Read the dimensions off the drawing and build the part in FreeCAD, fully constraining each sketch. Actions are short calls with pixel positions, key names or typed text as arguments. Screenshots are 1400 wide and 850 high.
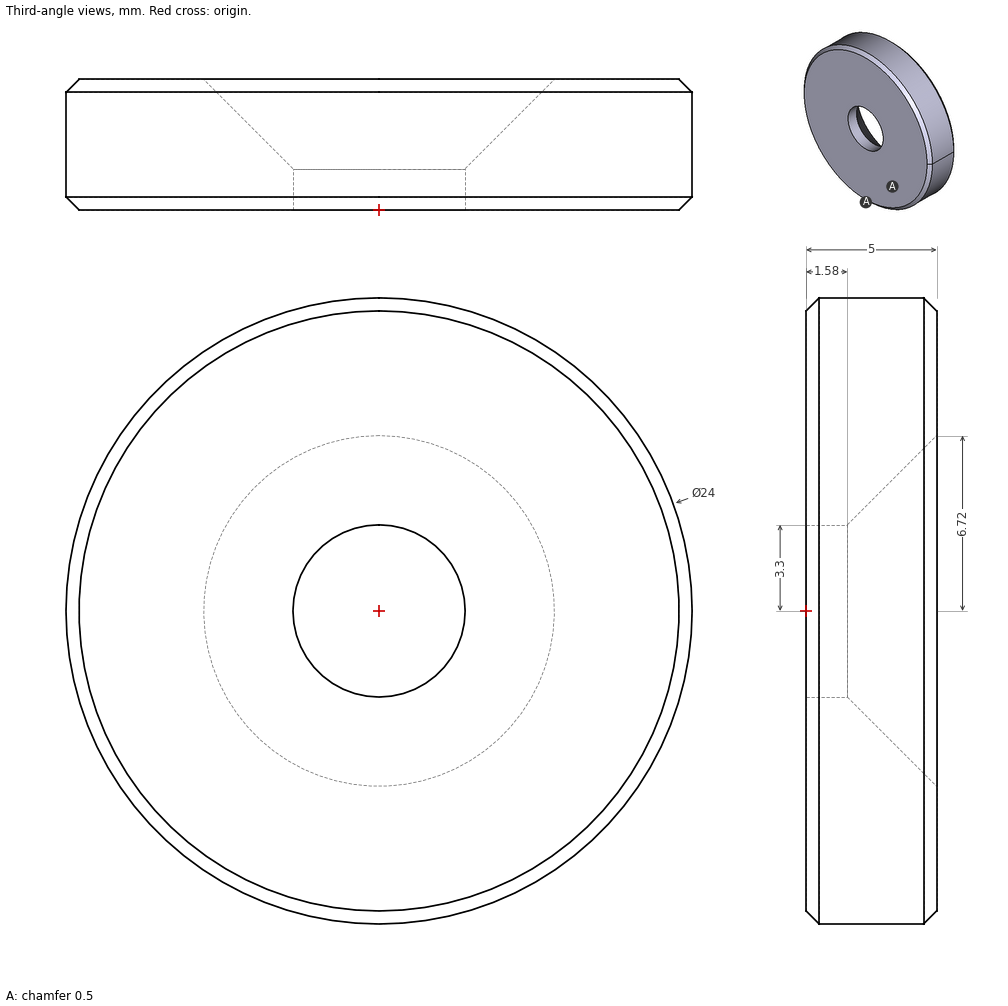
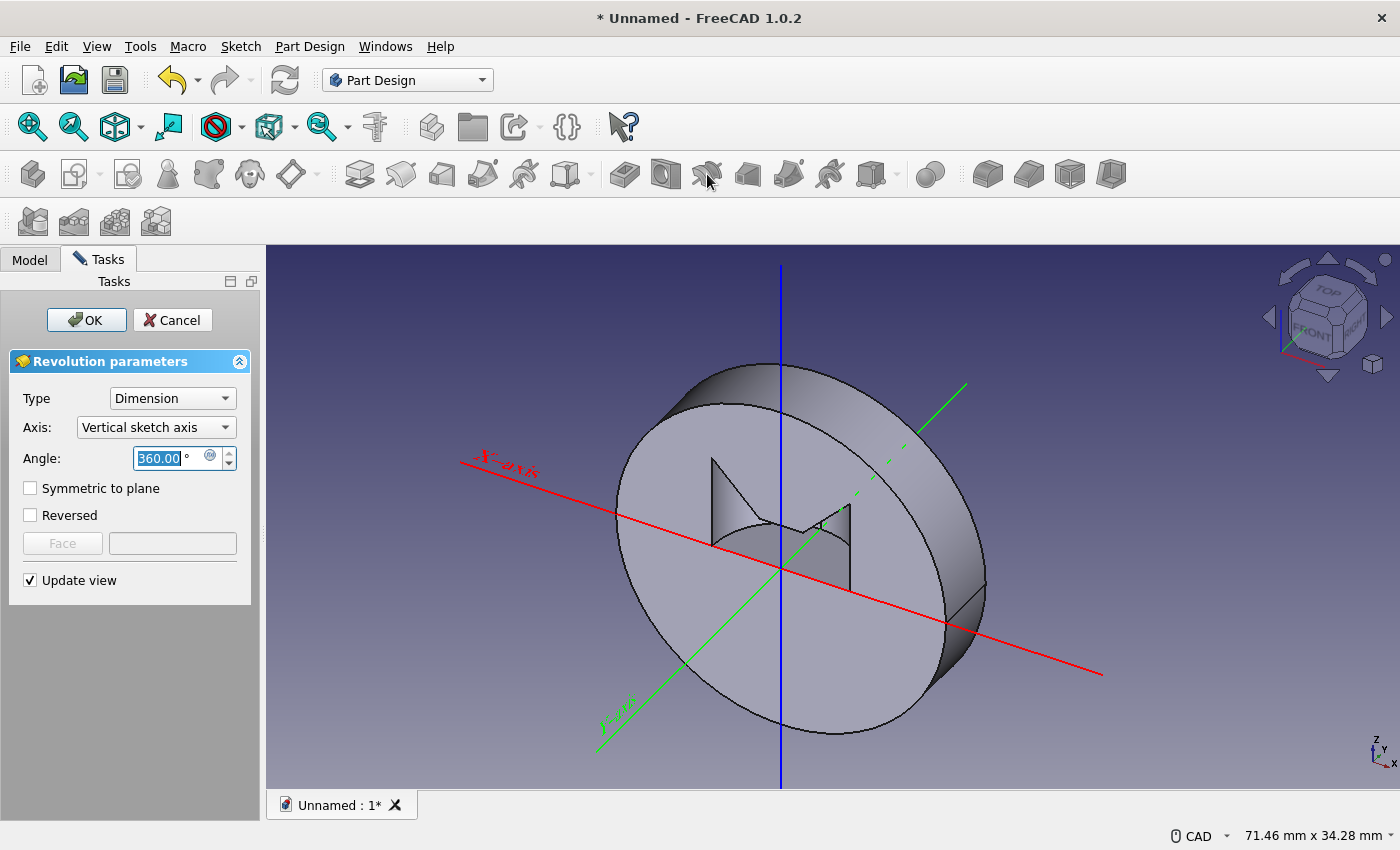
click(157, 428)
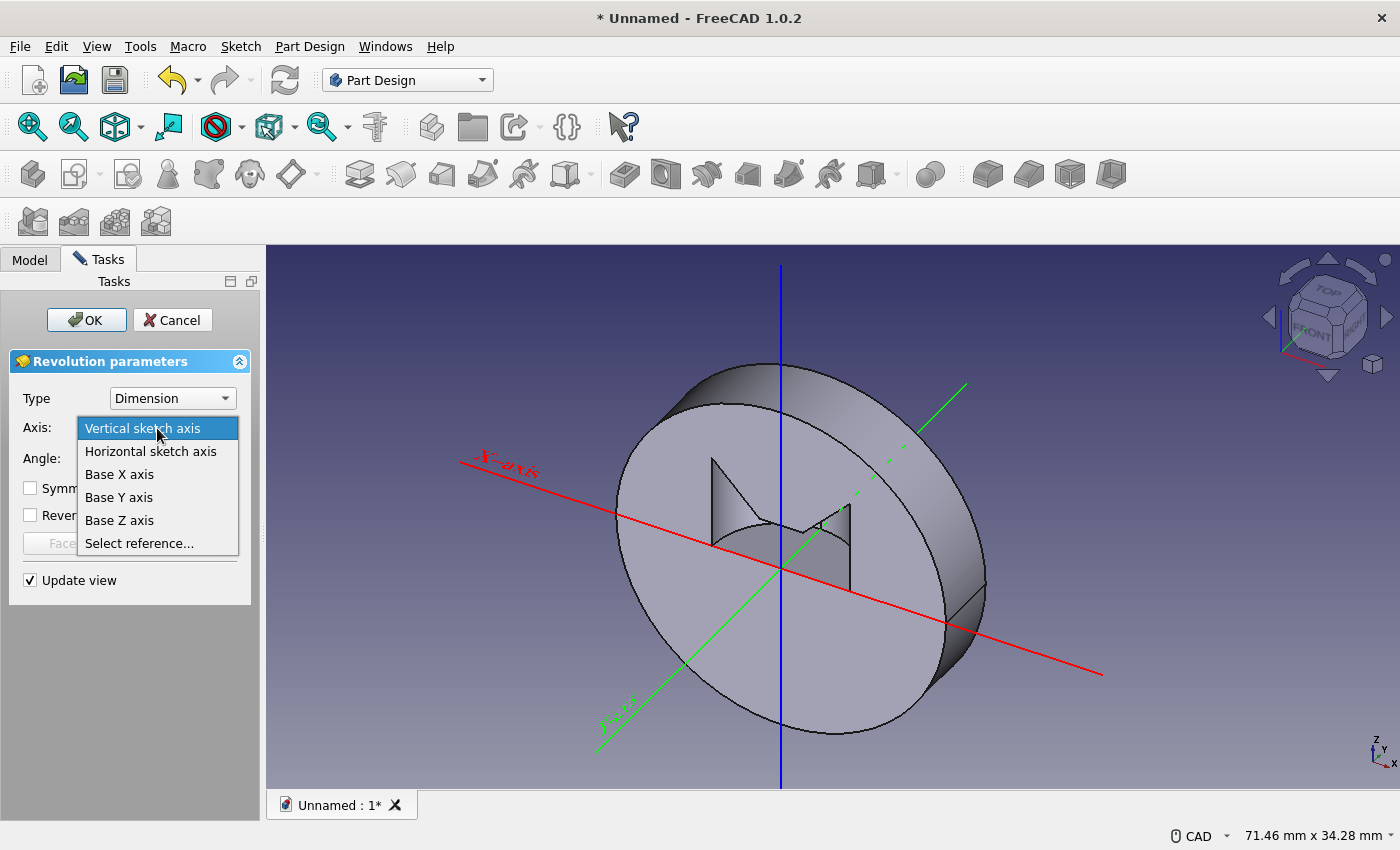
click(156, 452)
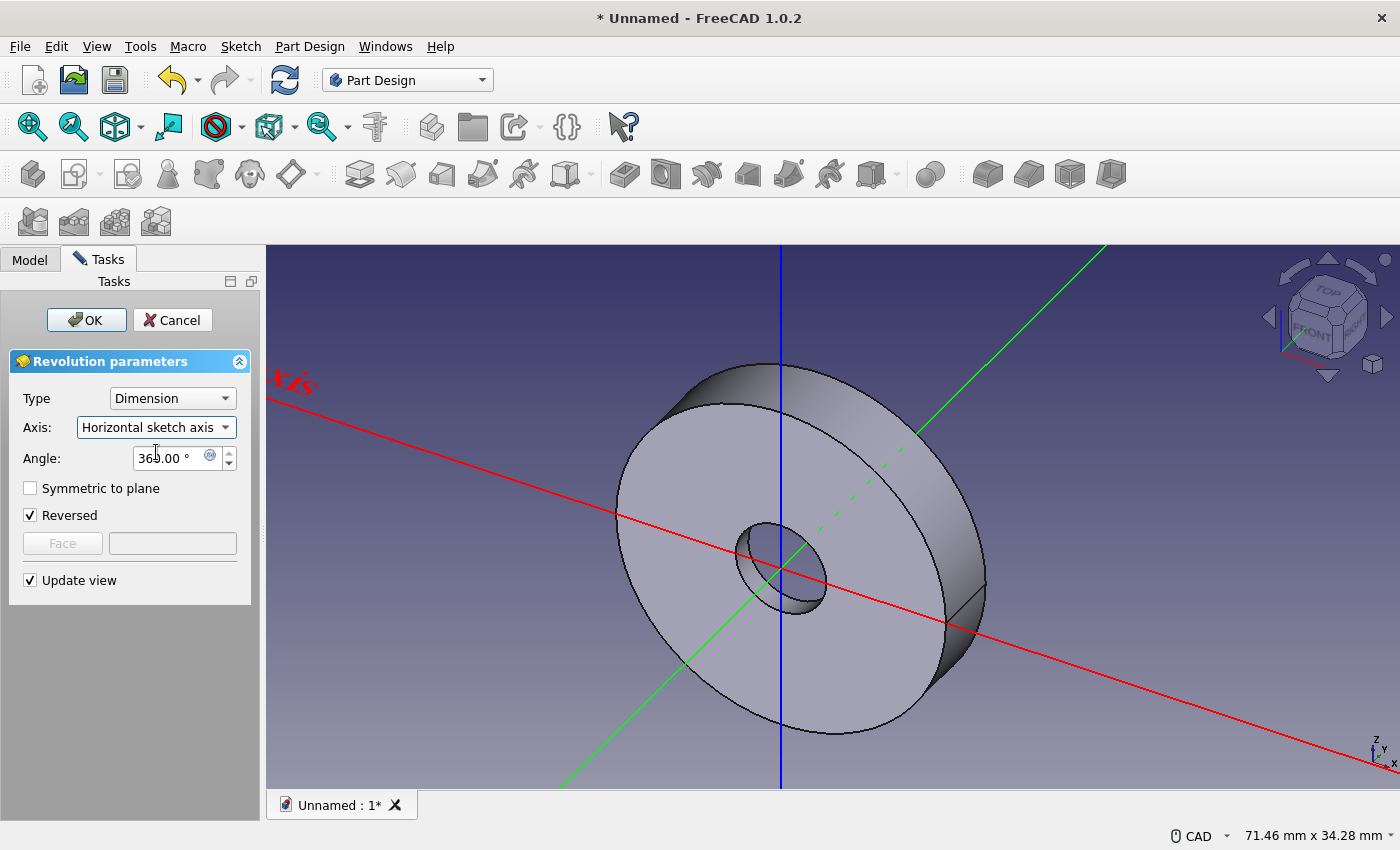
click(87, 320)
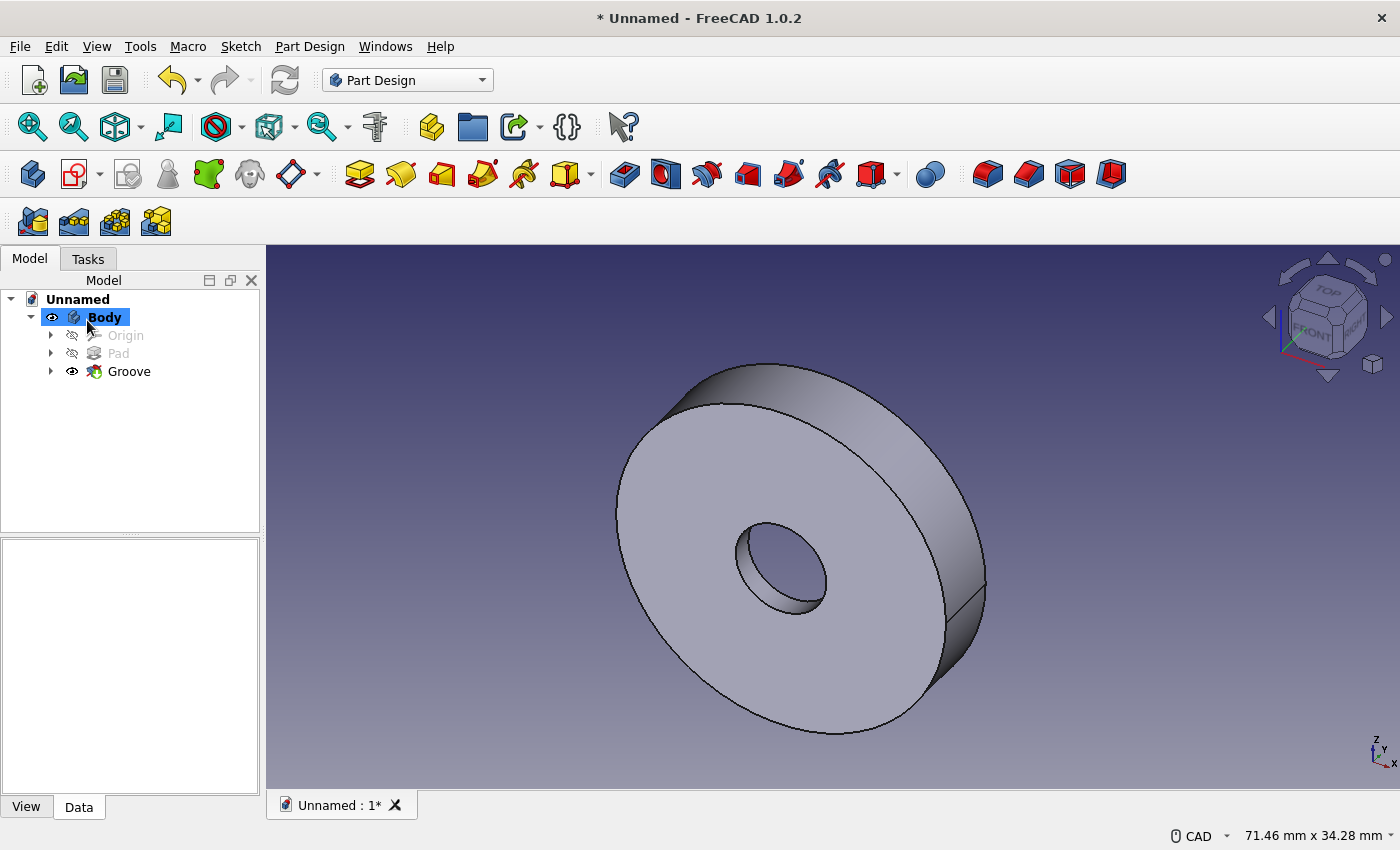
click(730, 402)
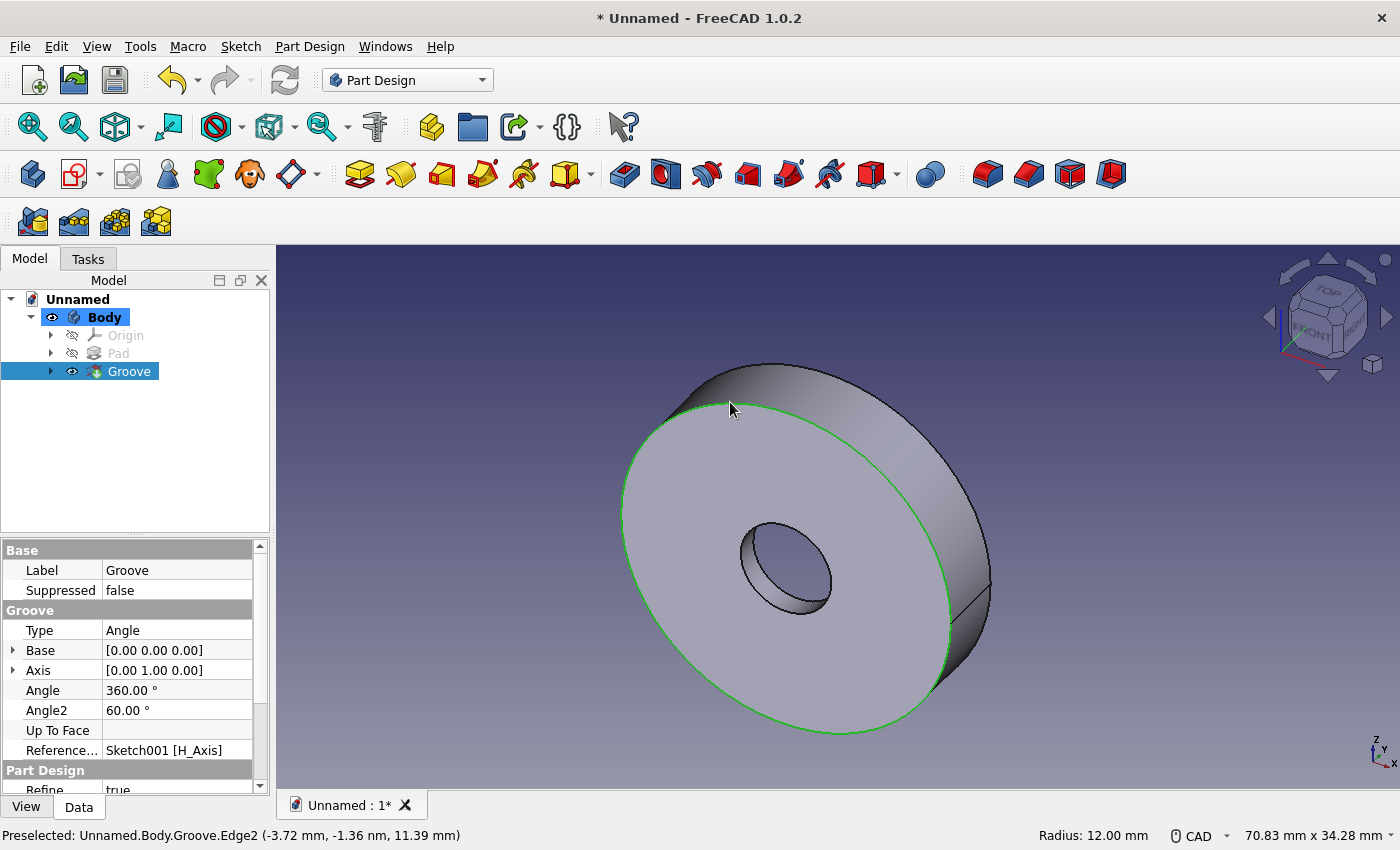
key(0)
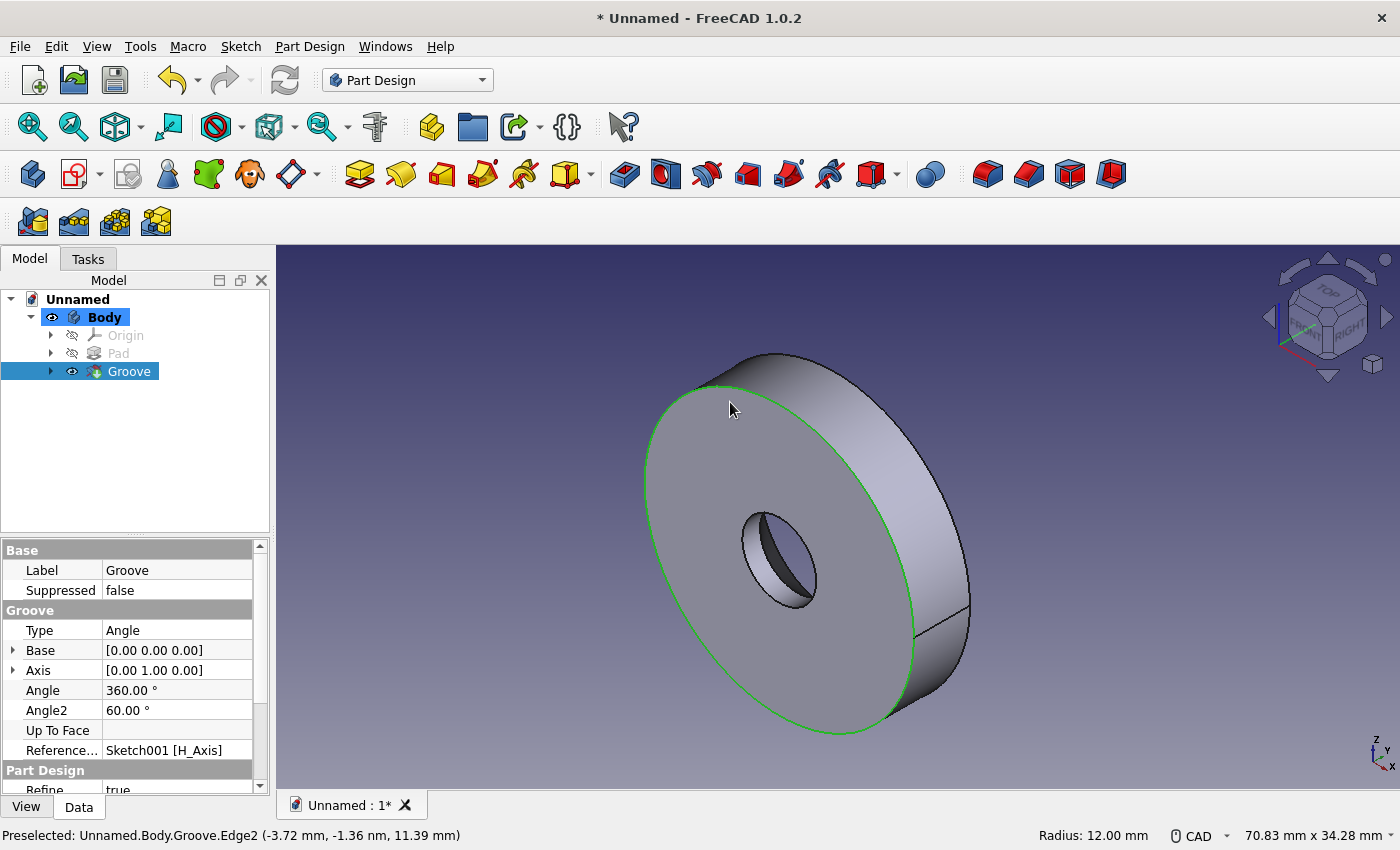
click(33, 128)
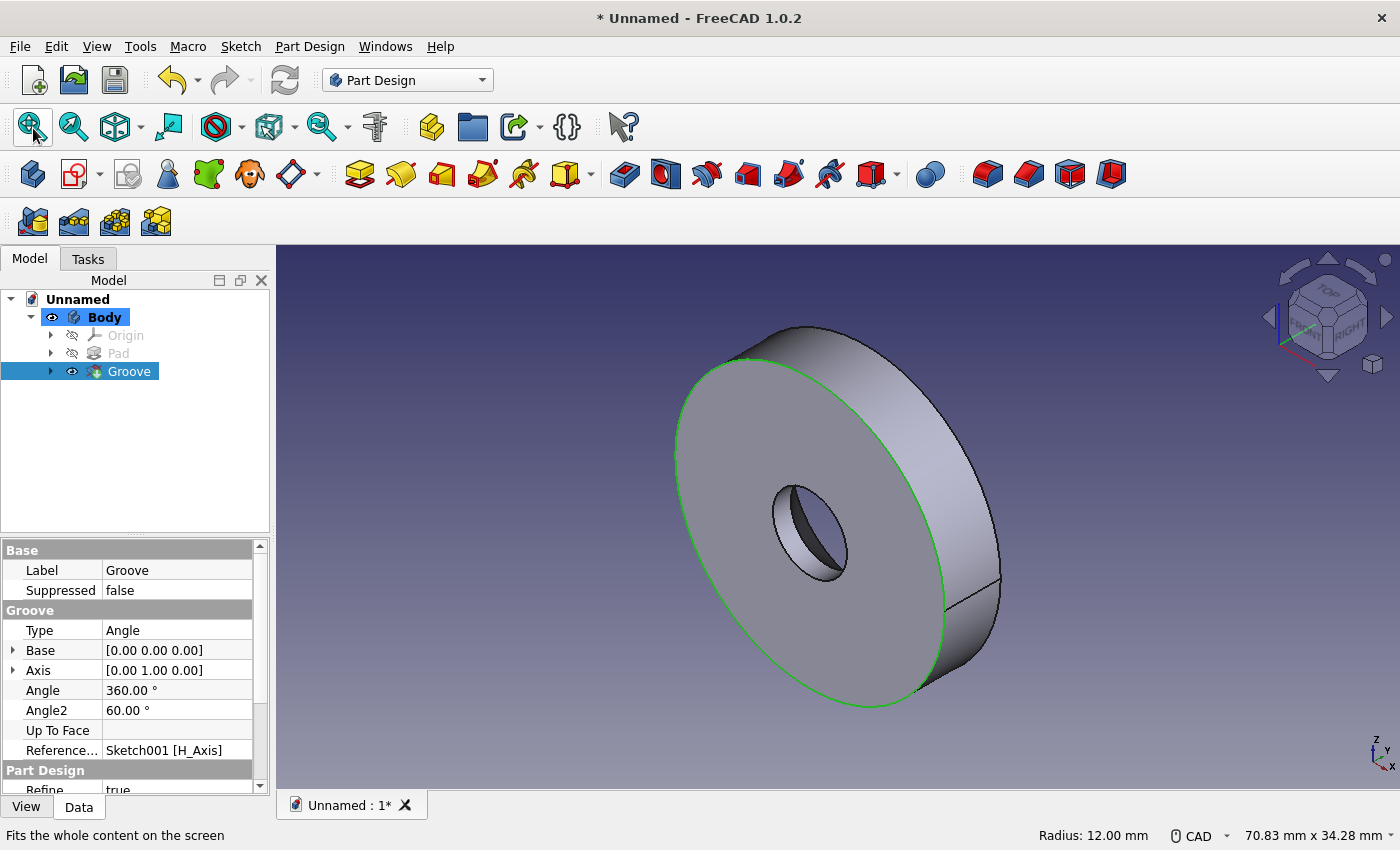
key(2)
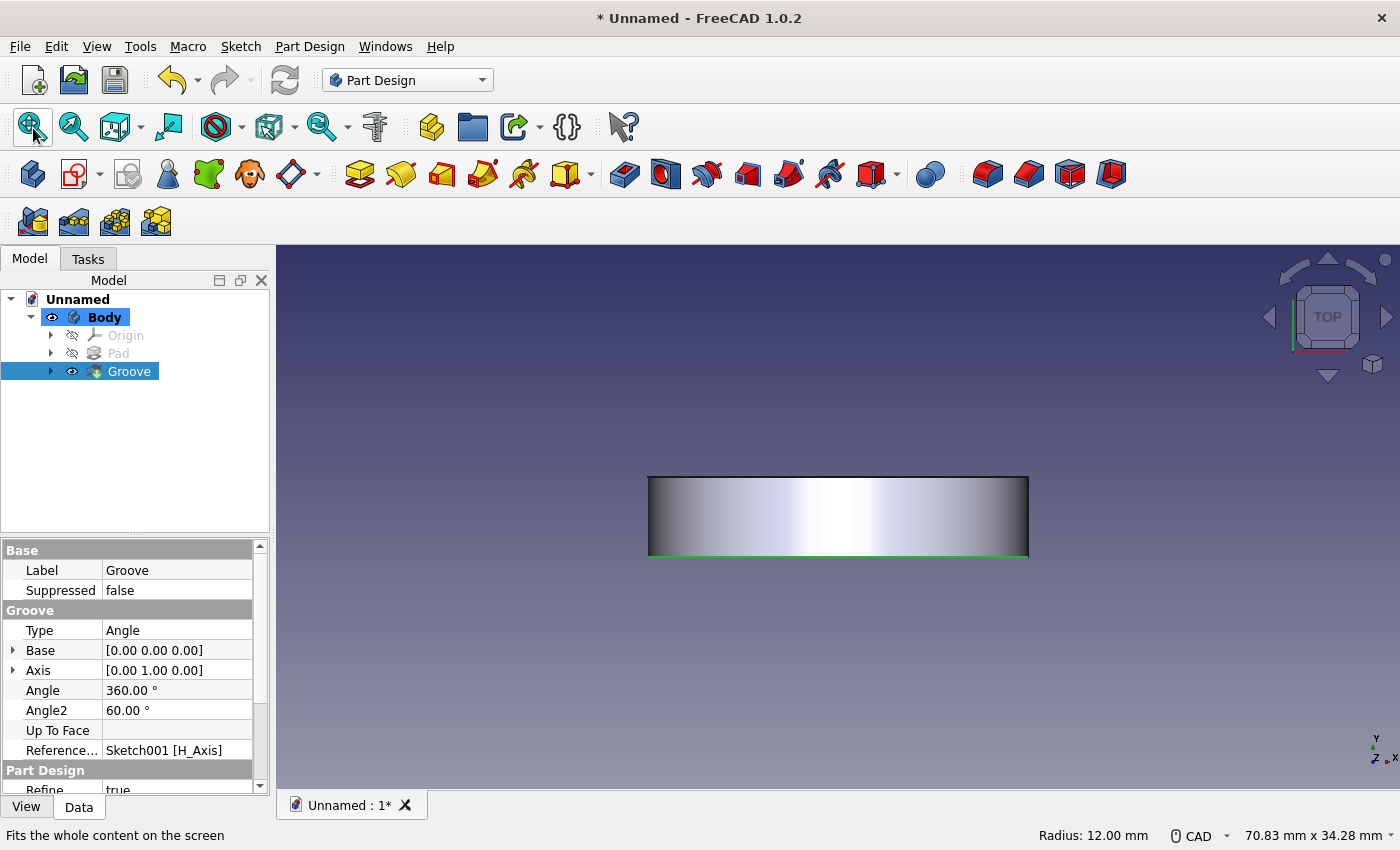
click(33, 128)